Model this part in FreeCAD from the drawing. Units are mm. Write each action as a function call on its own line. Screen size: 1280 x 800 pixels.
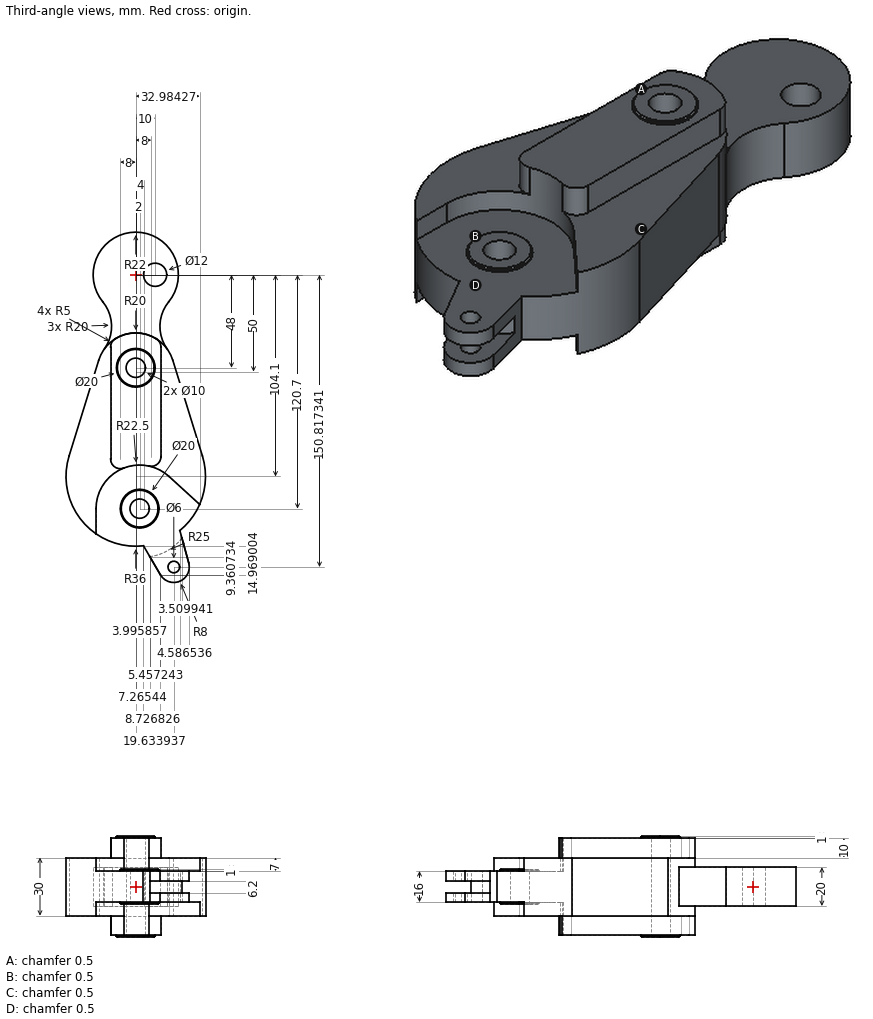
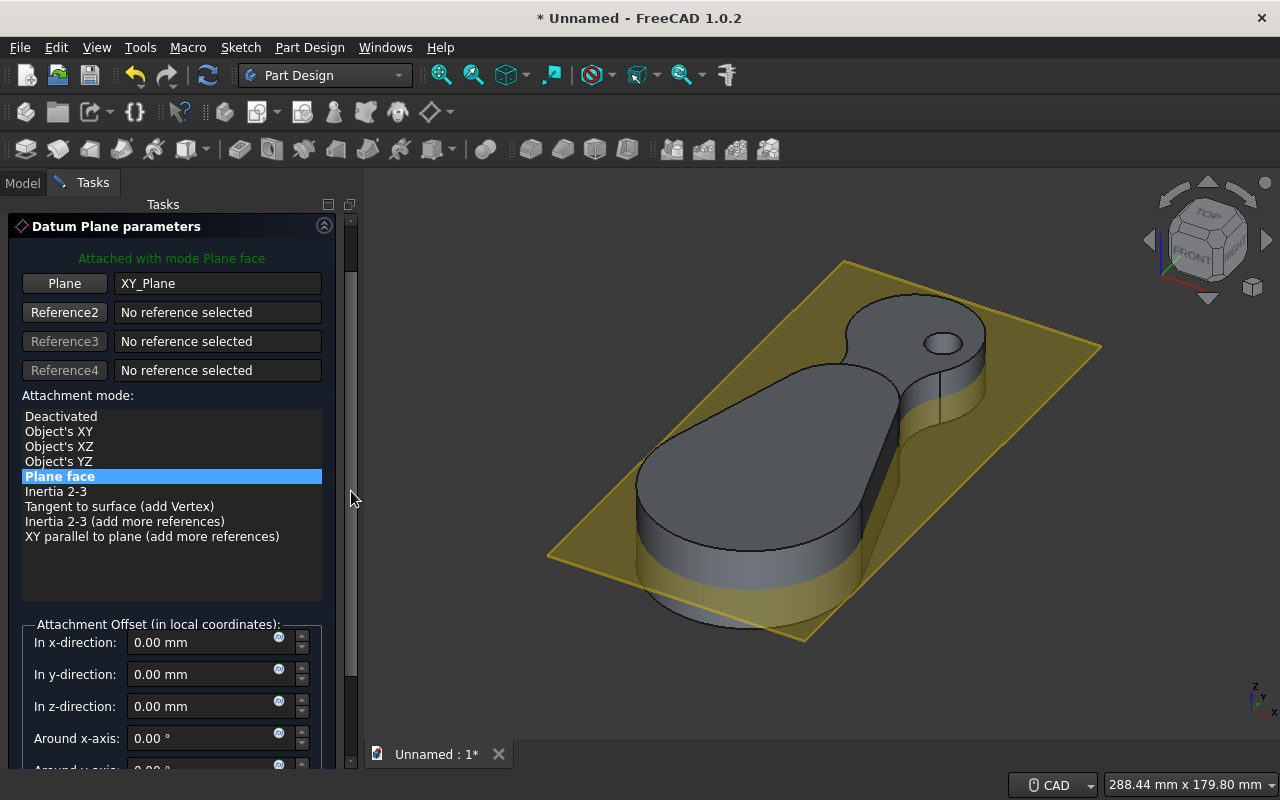
triple_click(210, 646)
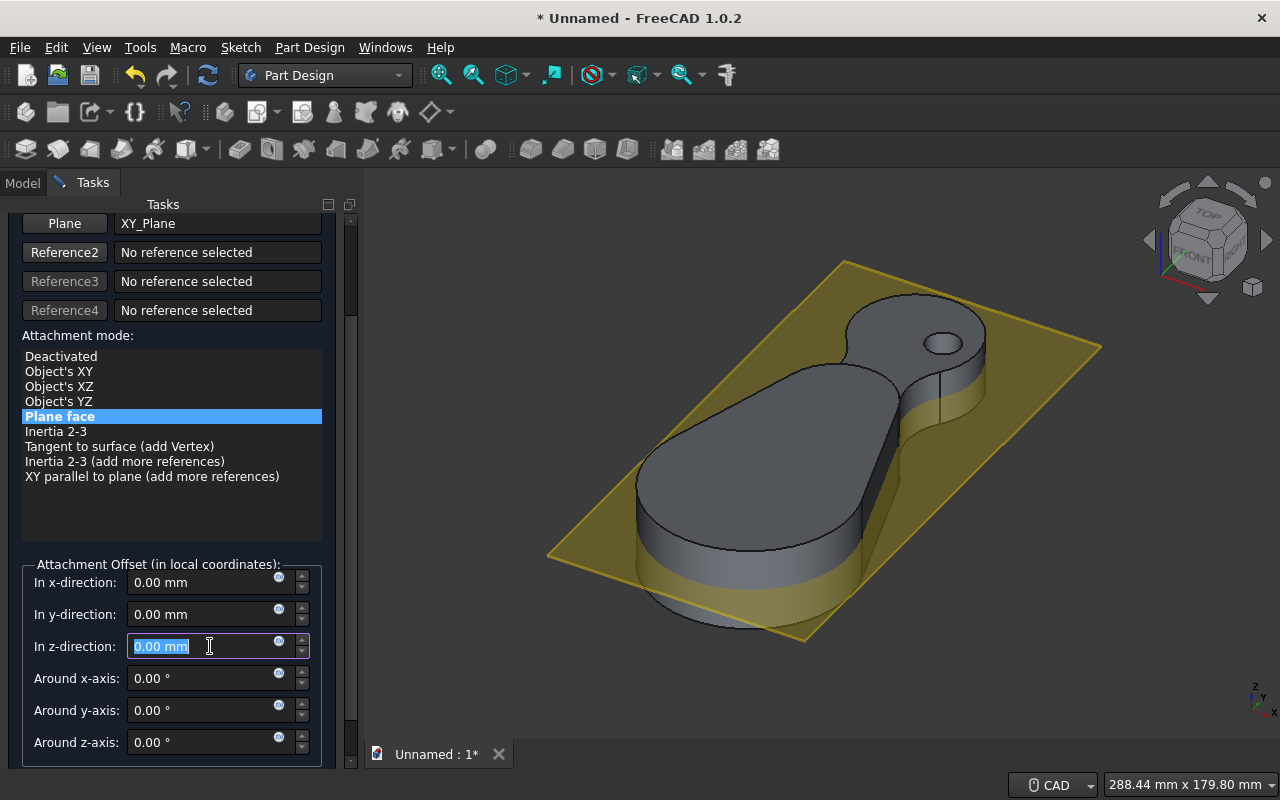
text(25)
key(Tab)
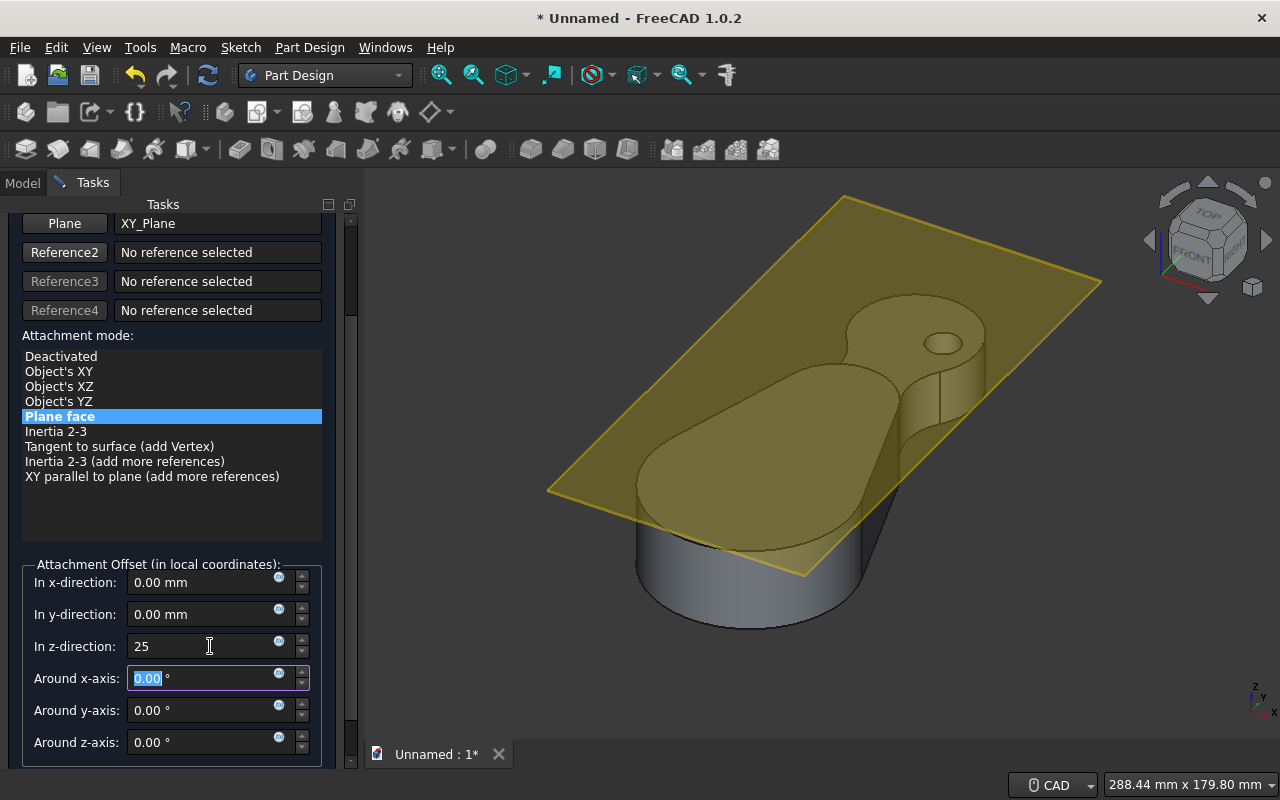
scroll(351, 491, up, 3)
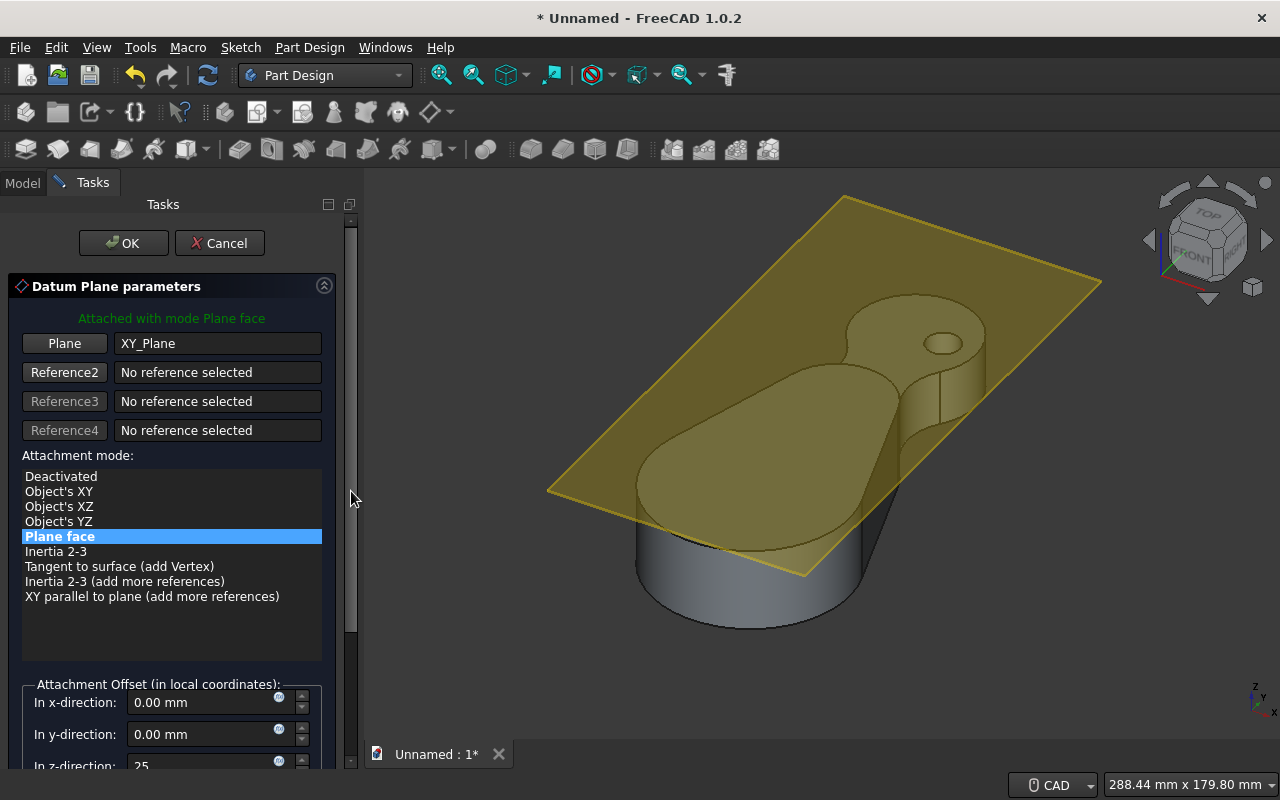
click(124, 243)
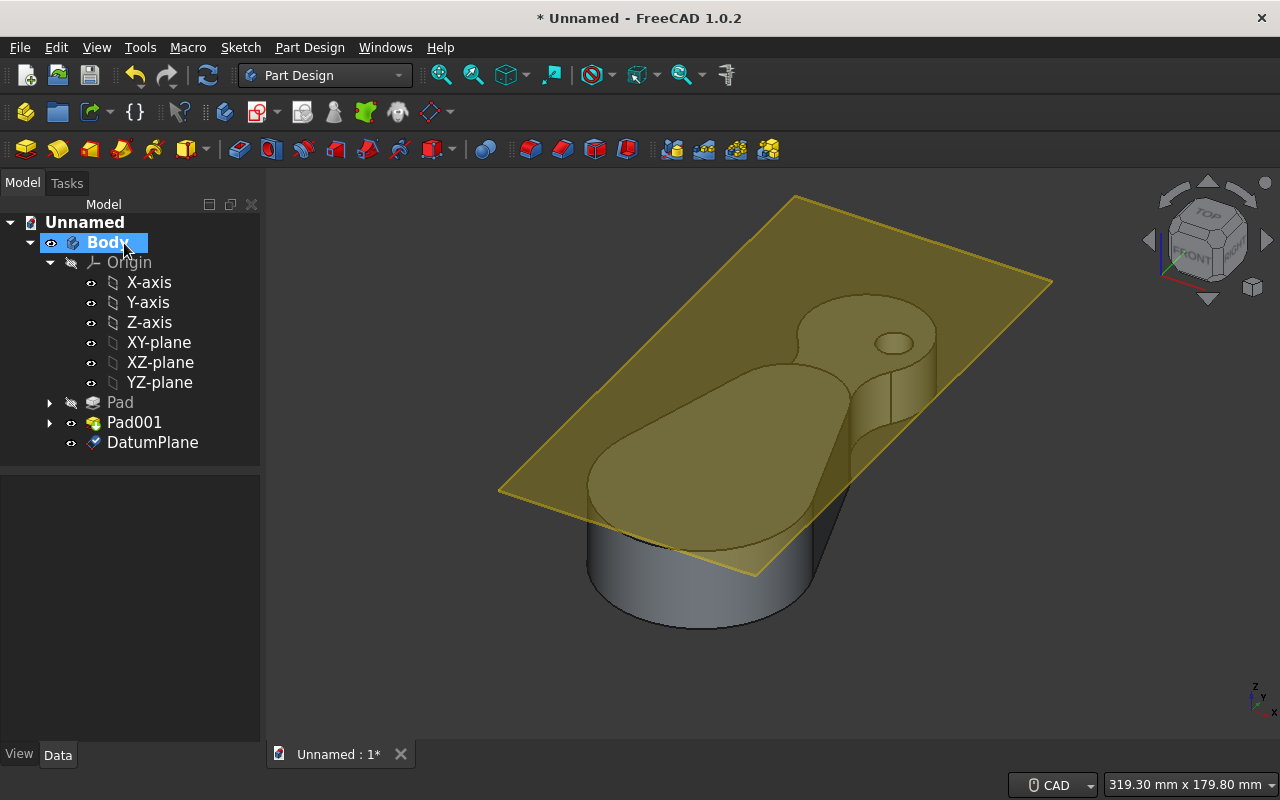
click(116, 443)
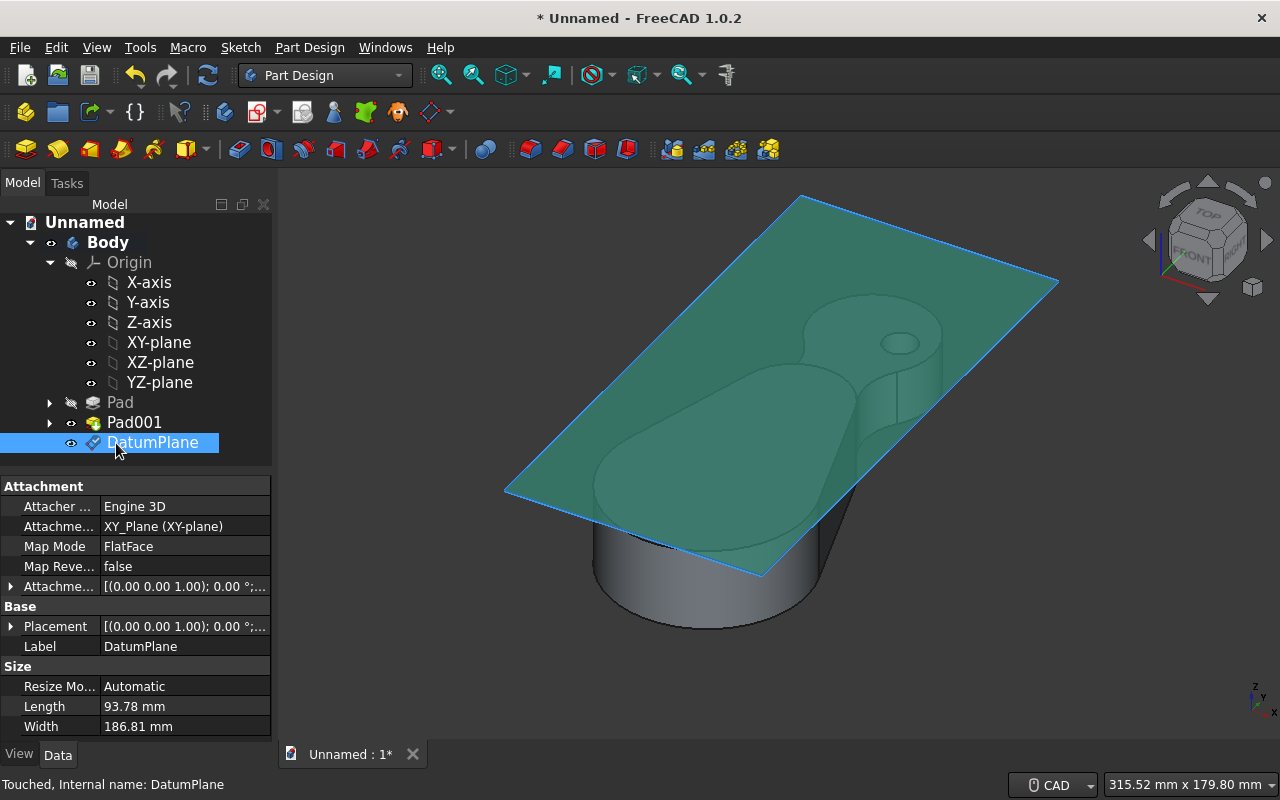
click(258, 112)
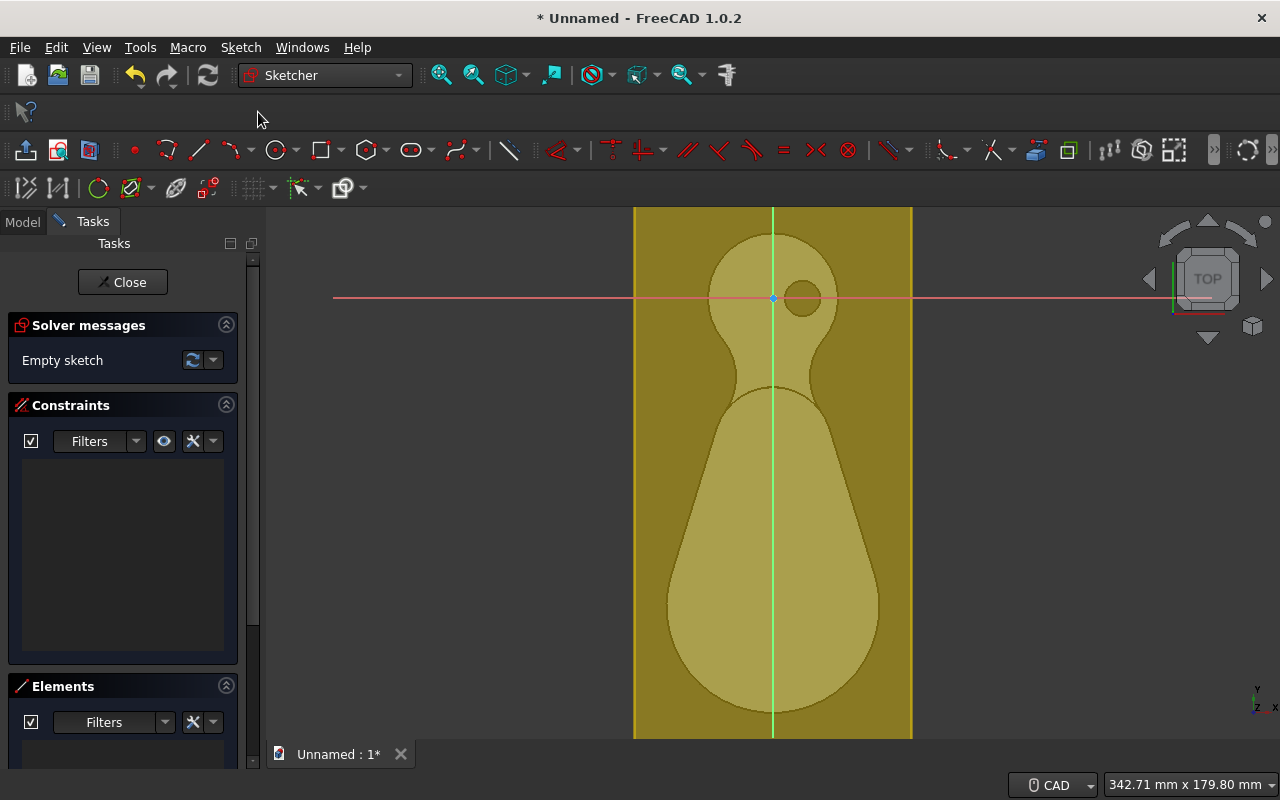
click(200, 150)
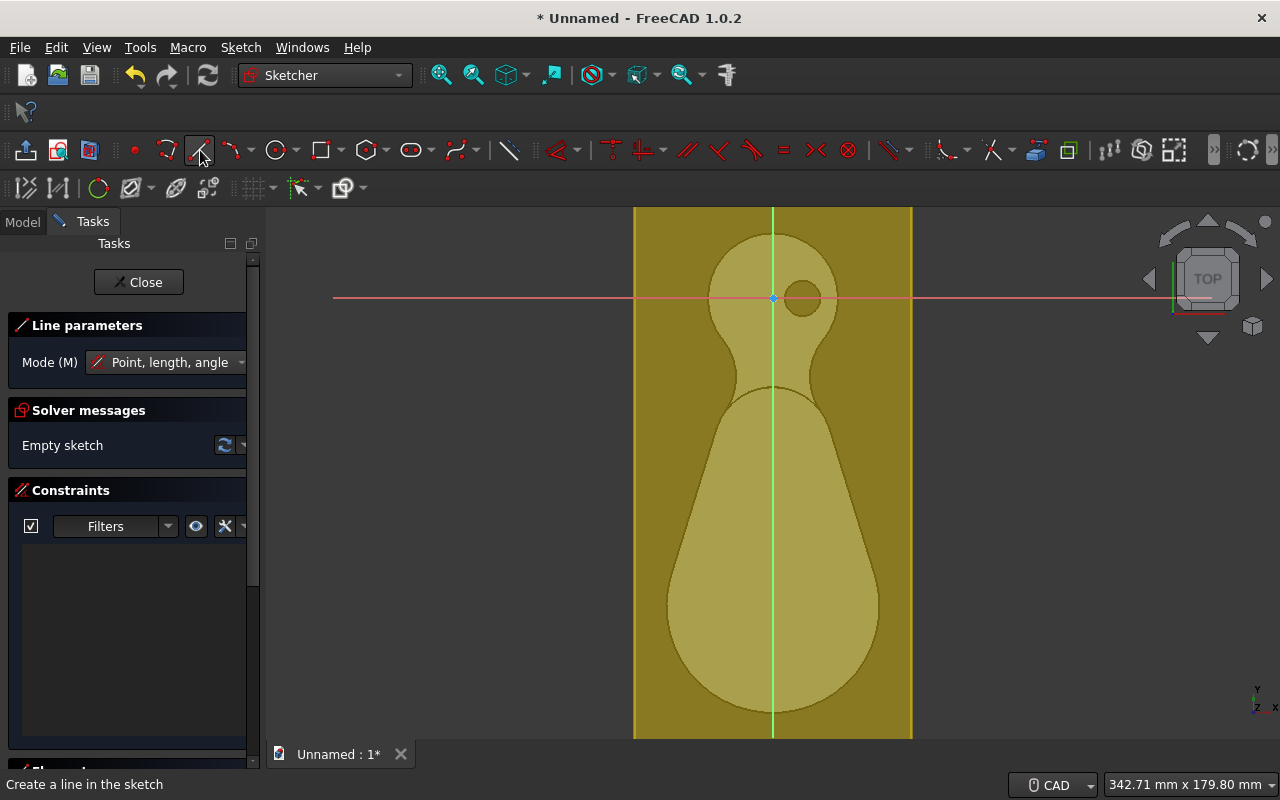
click(735, 409)
click(735, 580)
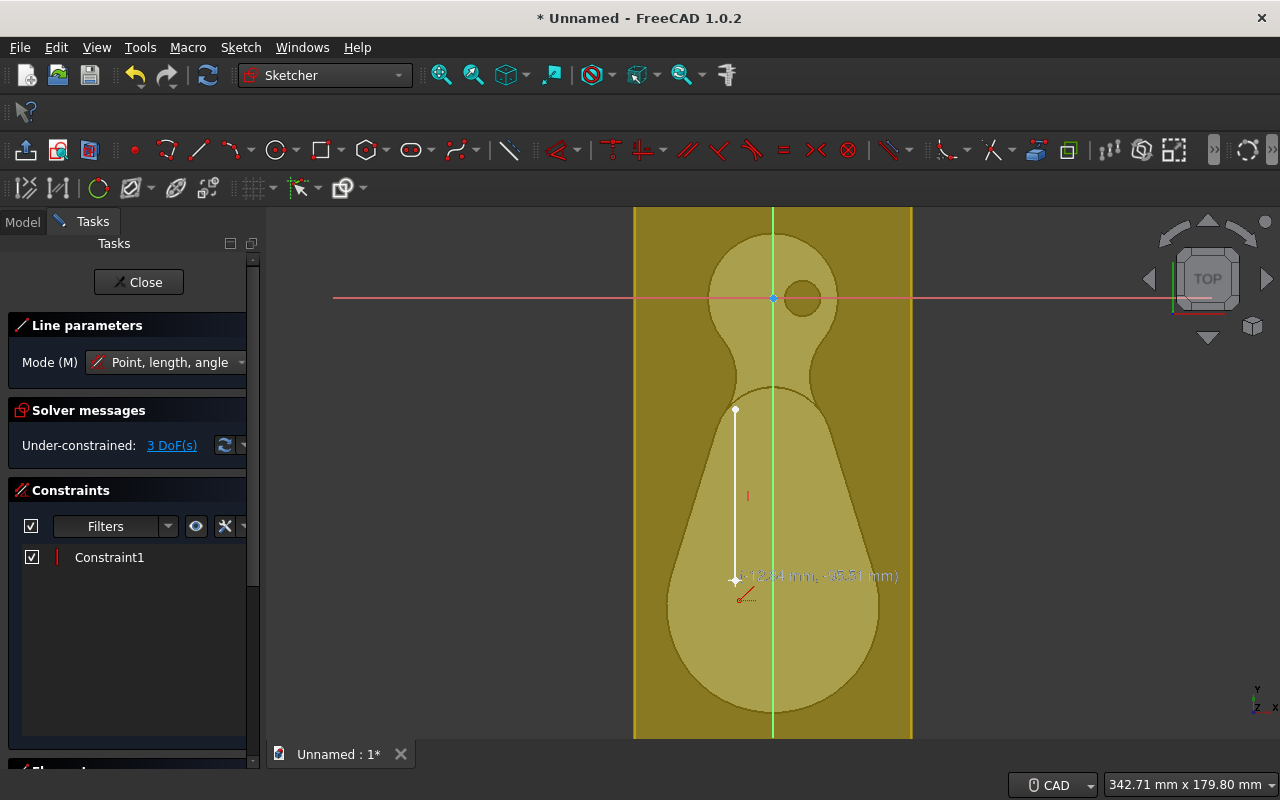
click(811, 576)
click(811, 409)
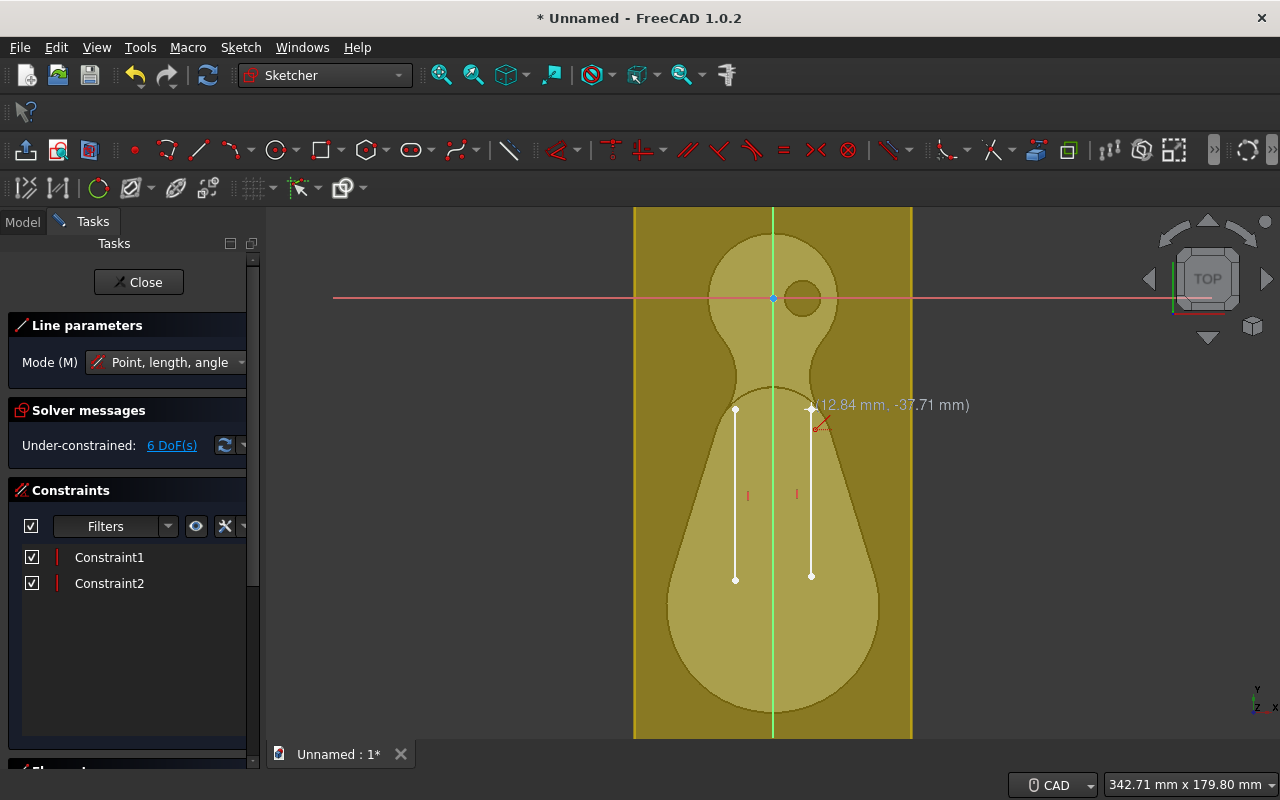
click(232, 150)